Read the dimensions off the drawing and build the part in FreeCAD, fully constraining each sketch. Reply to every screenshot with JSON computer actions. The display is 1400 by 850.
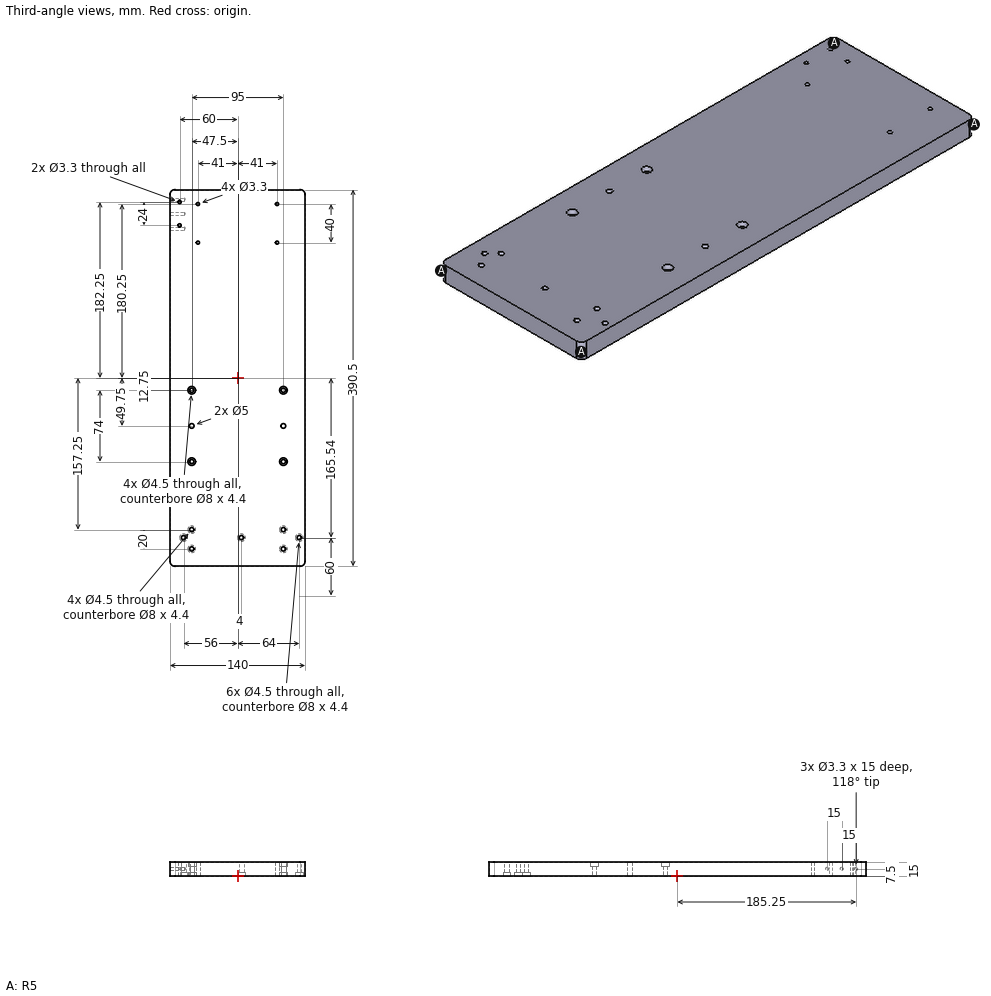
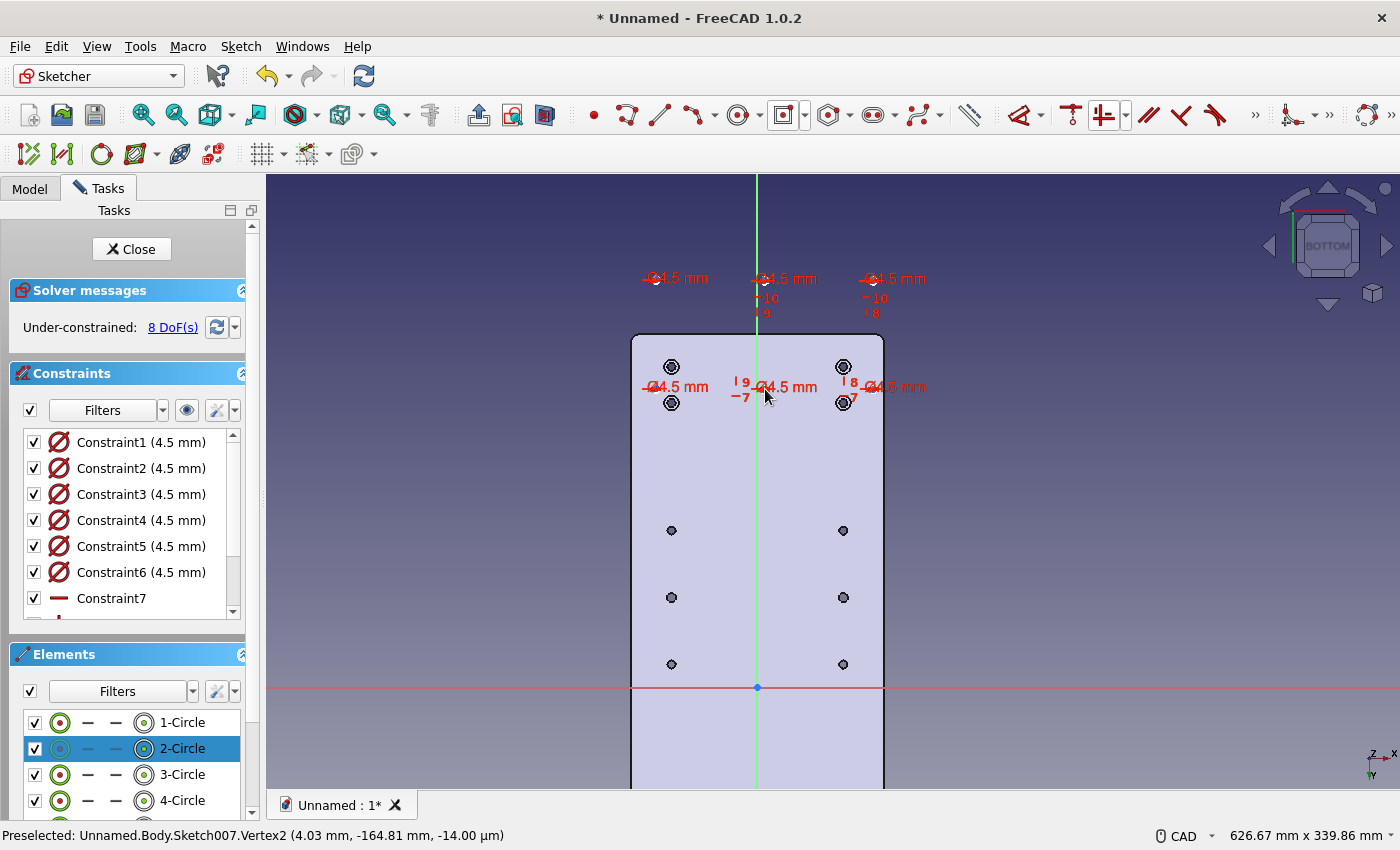
{"action": "left_click", "coordinate": [656, 389]}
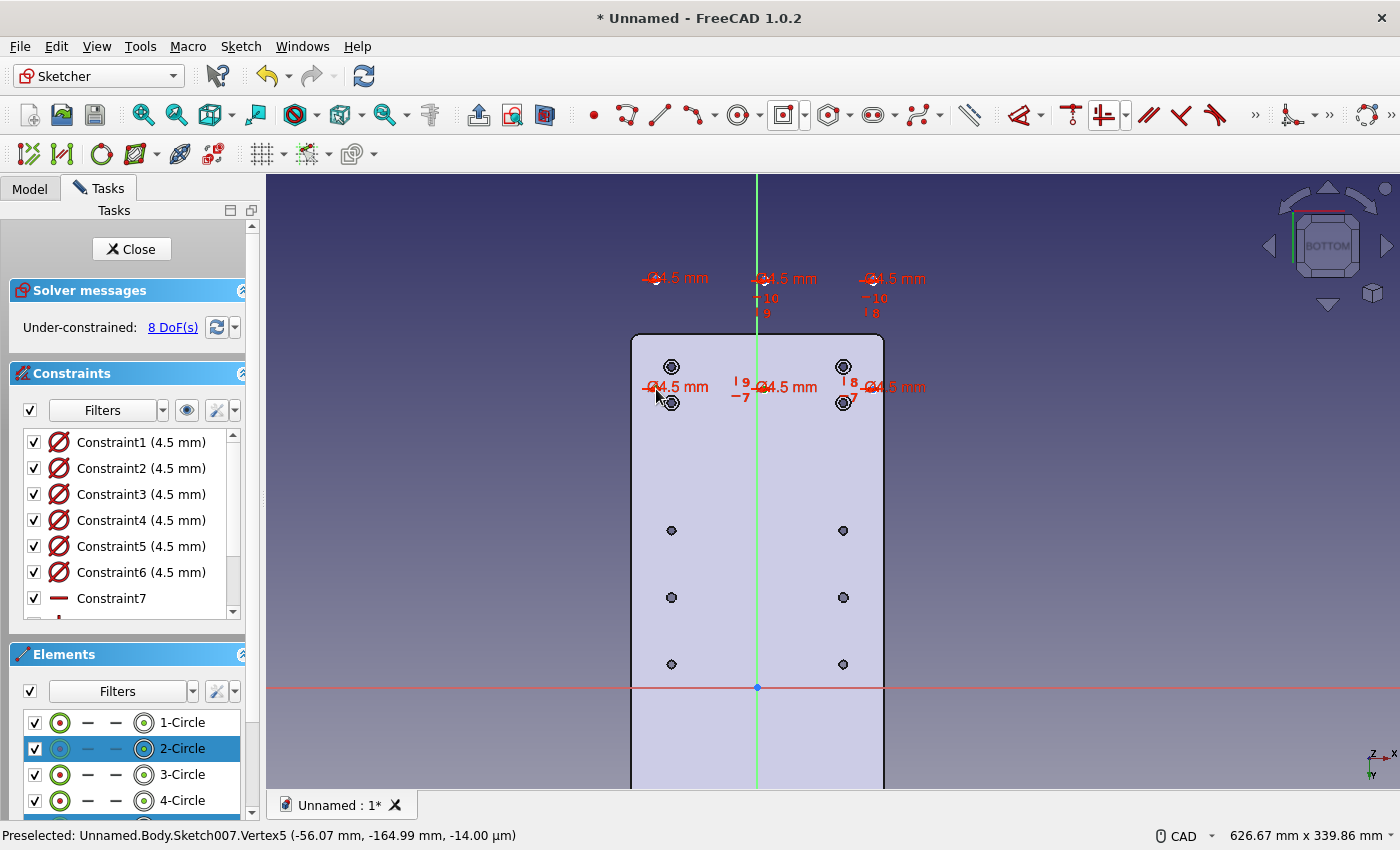
{"action": "left_click", "coordinate": [1126, 116]}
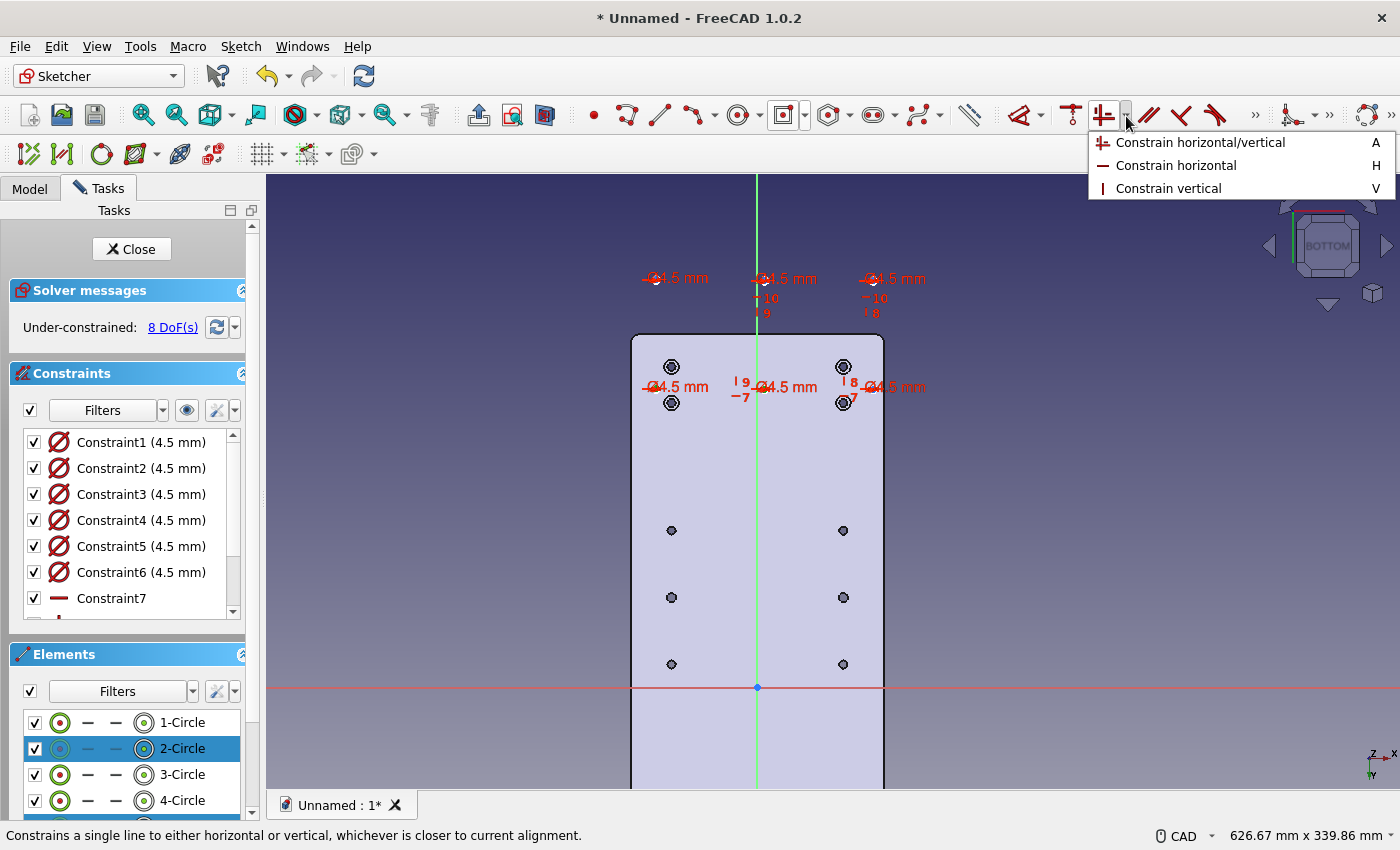
{"action": "left_click", "coordinate": [1242, 166]}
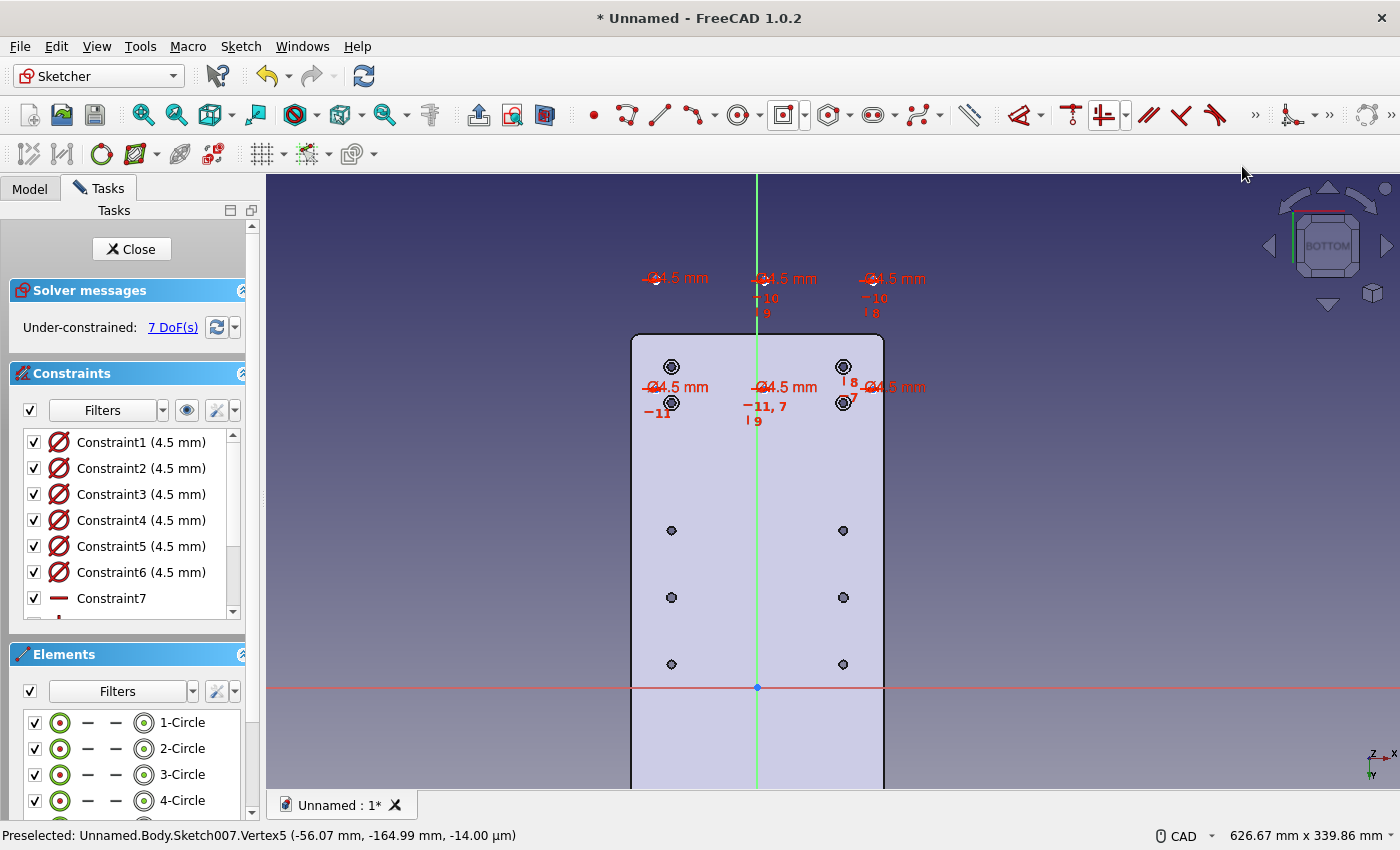
{"action": "left_click", "coordinate": [656, 389]}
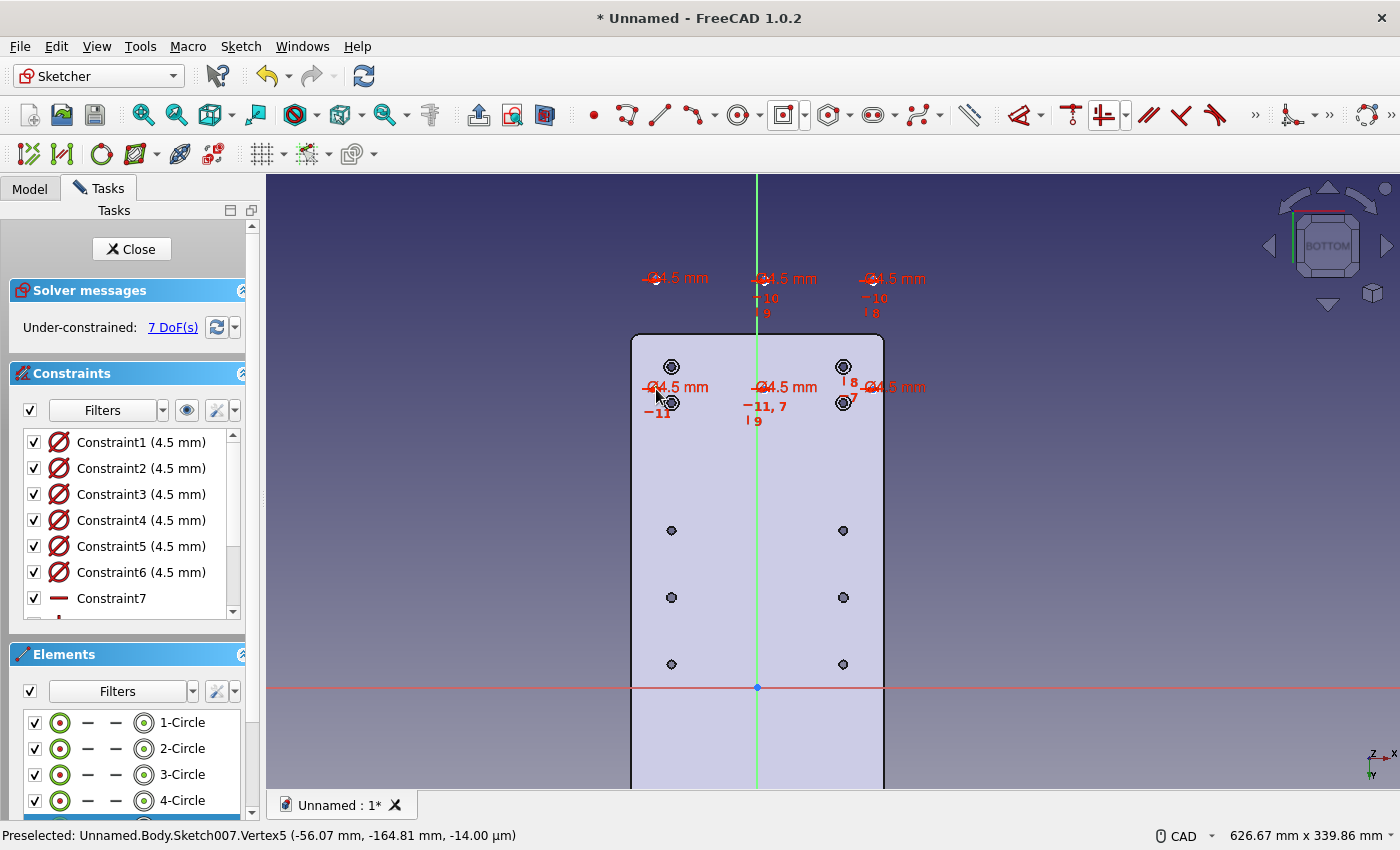
{"action": "left_click", "coordinate": [656, 280]}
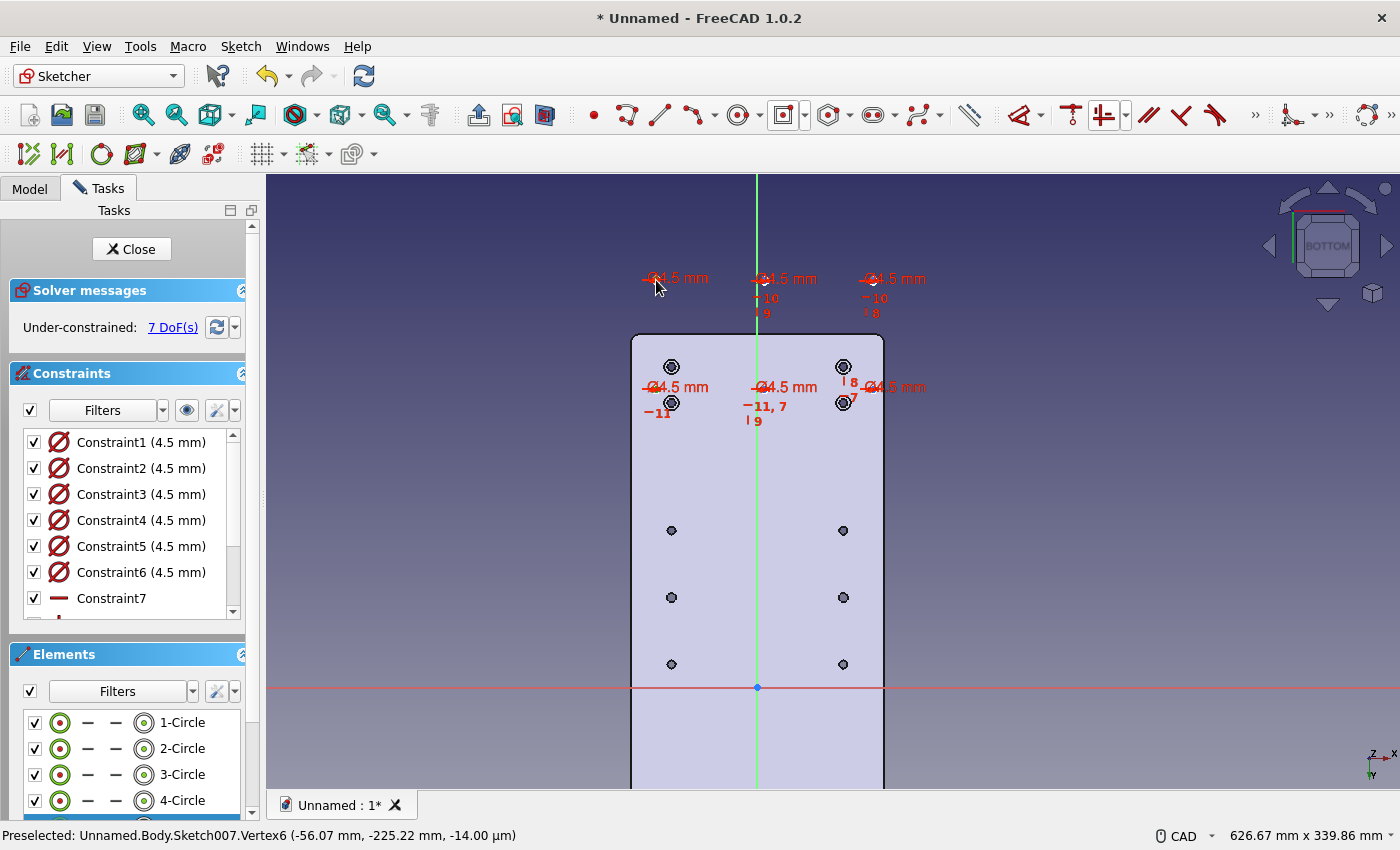
{"action": "key", "text": "v"}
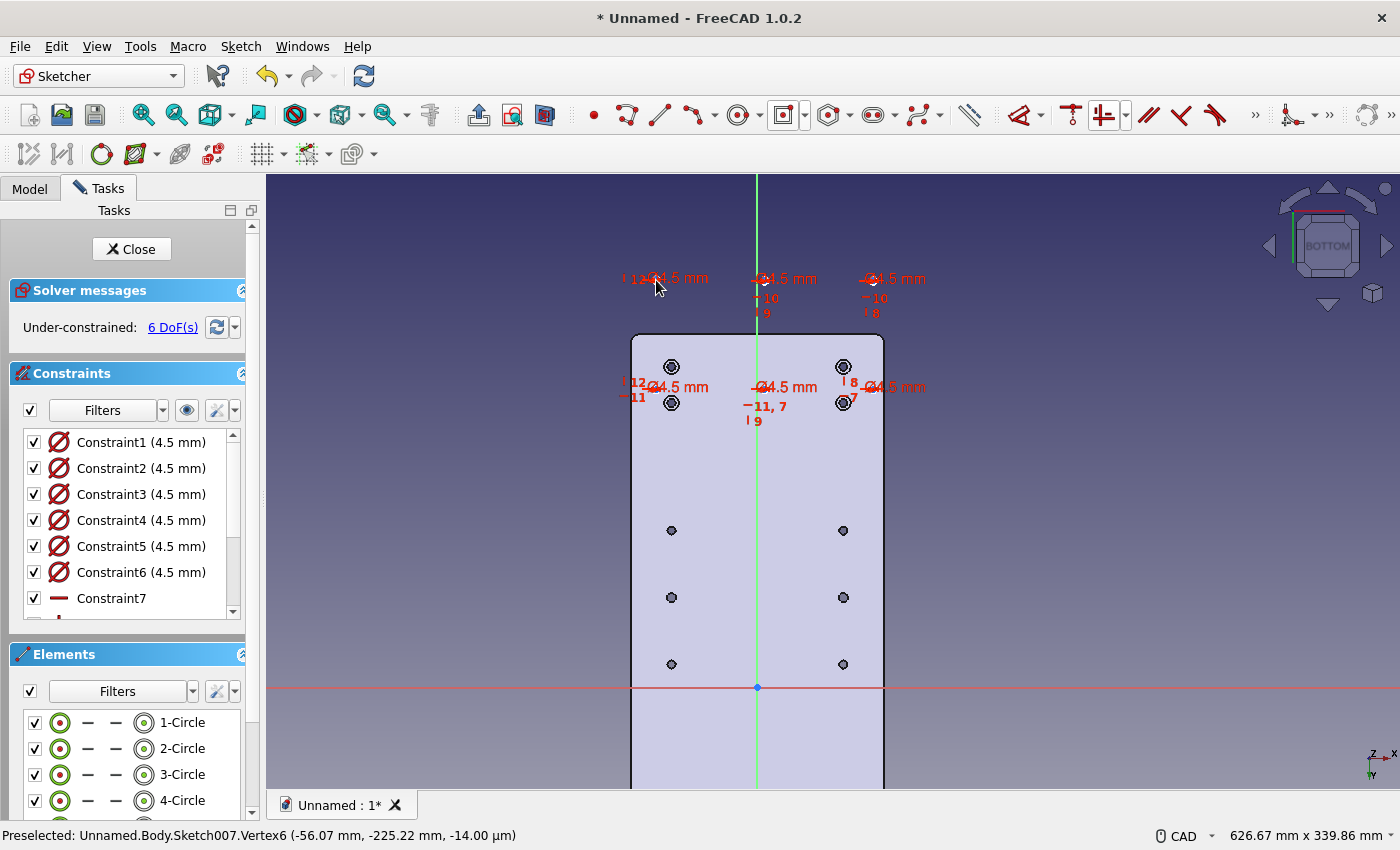
{"action": "left_click", "coordinate": [765, 281]}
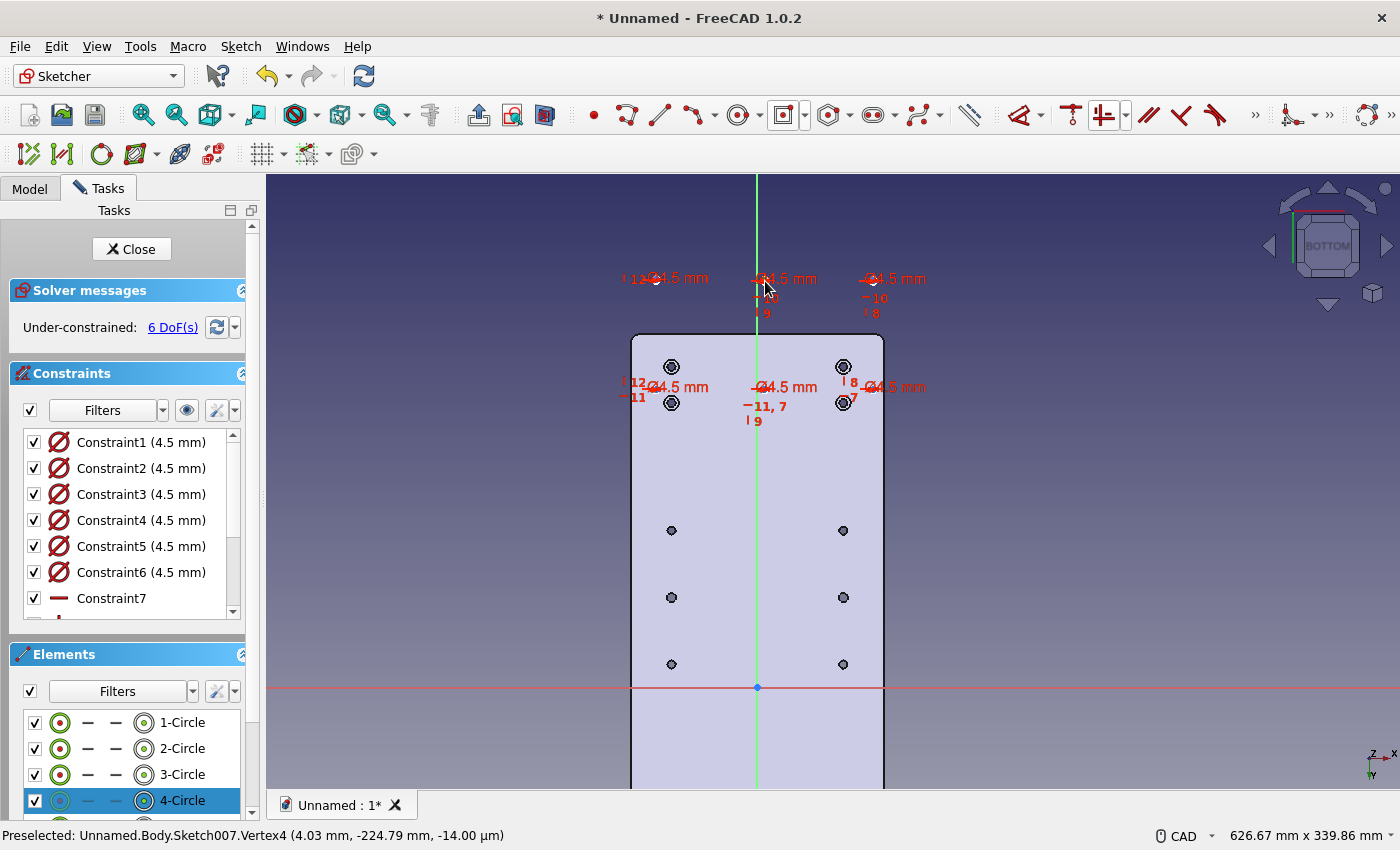
{"action": "left_click", "coordinate": [656, 280]}